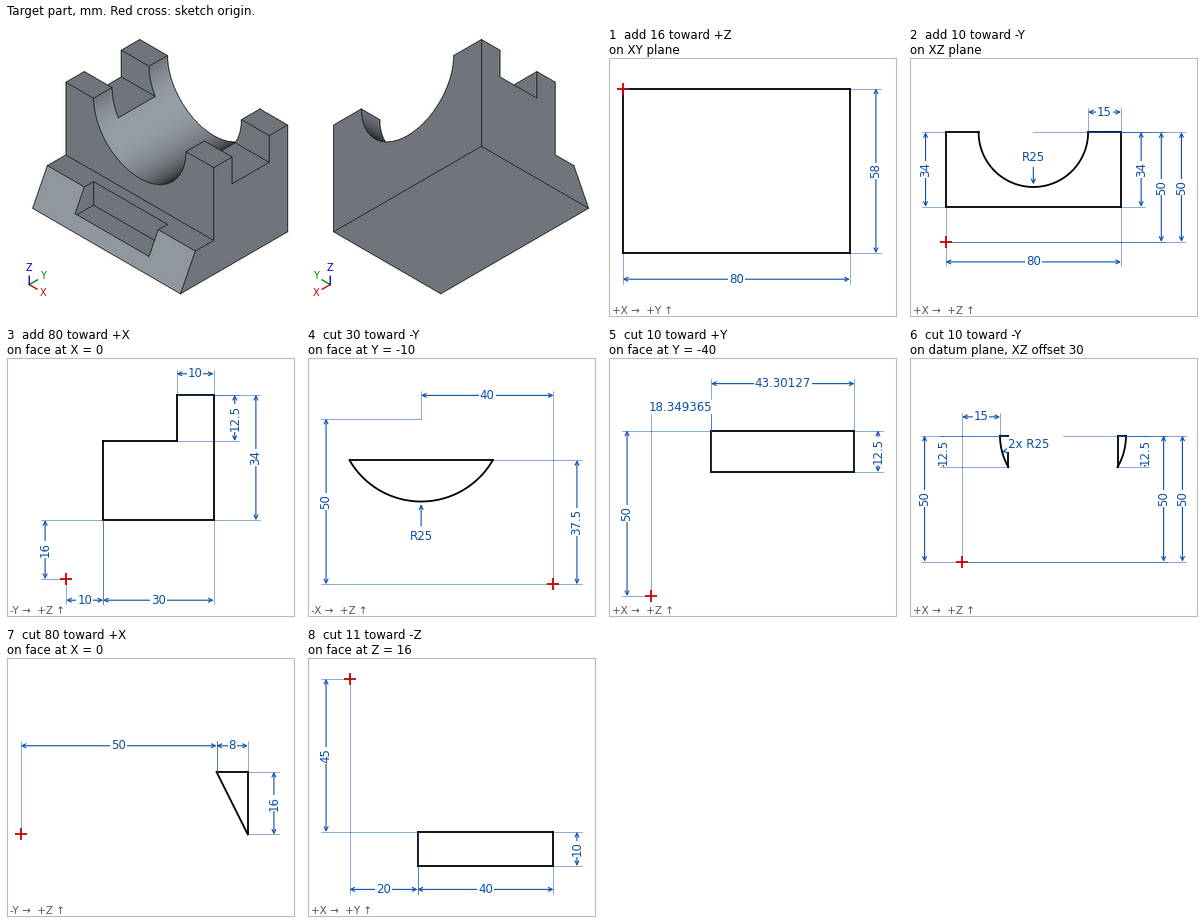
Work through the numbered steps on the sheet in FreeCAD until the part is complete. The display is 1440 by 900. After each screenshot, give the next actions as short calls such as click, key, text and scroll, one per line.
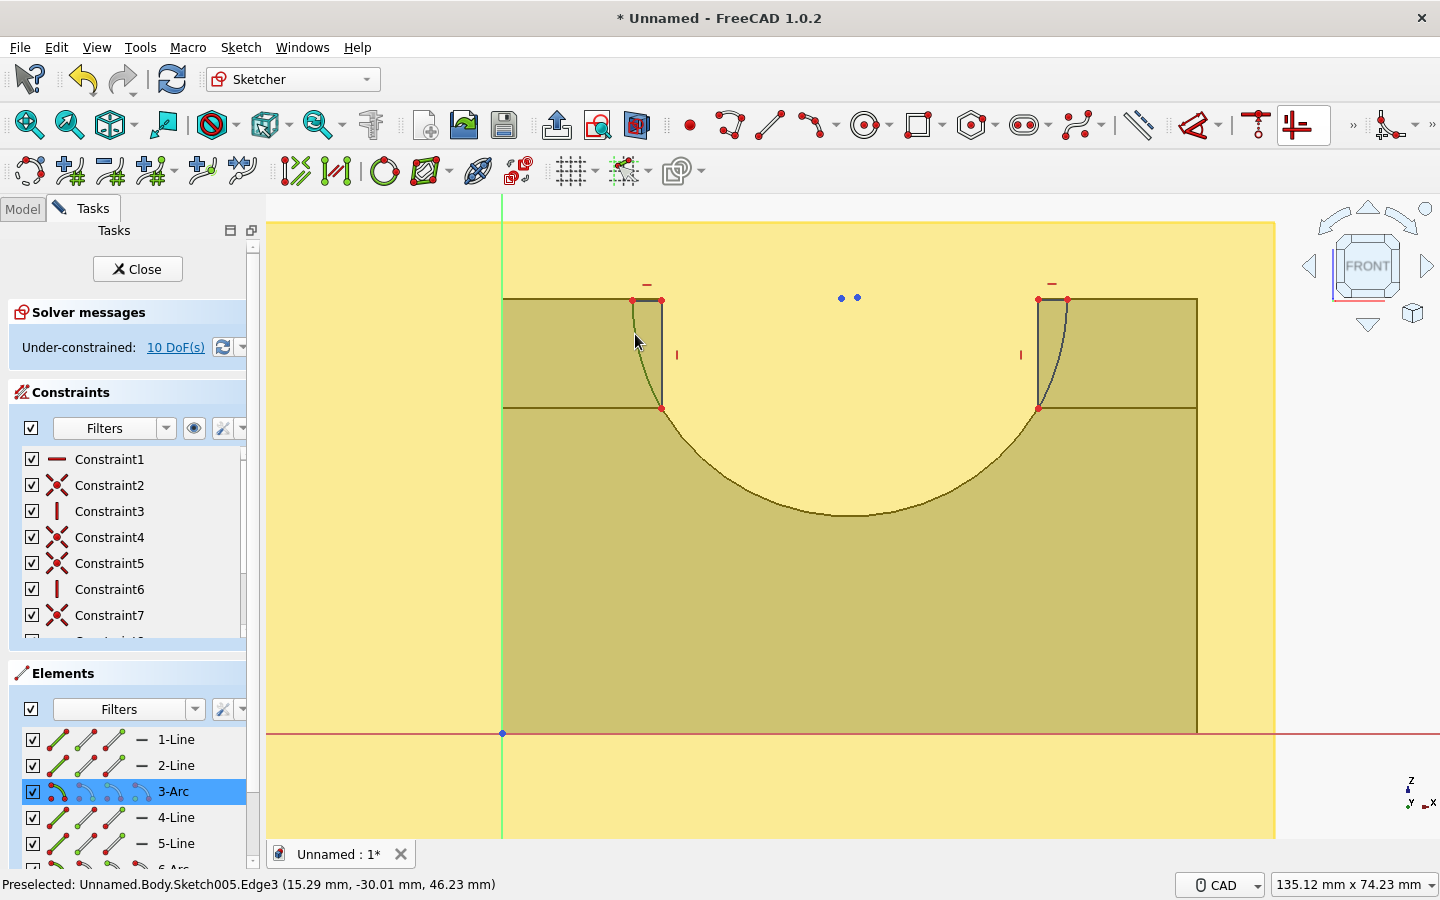
click(1052, 378)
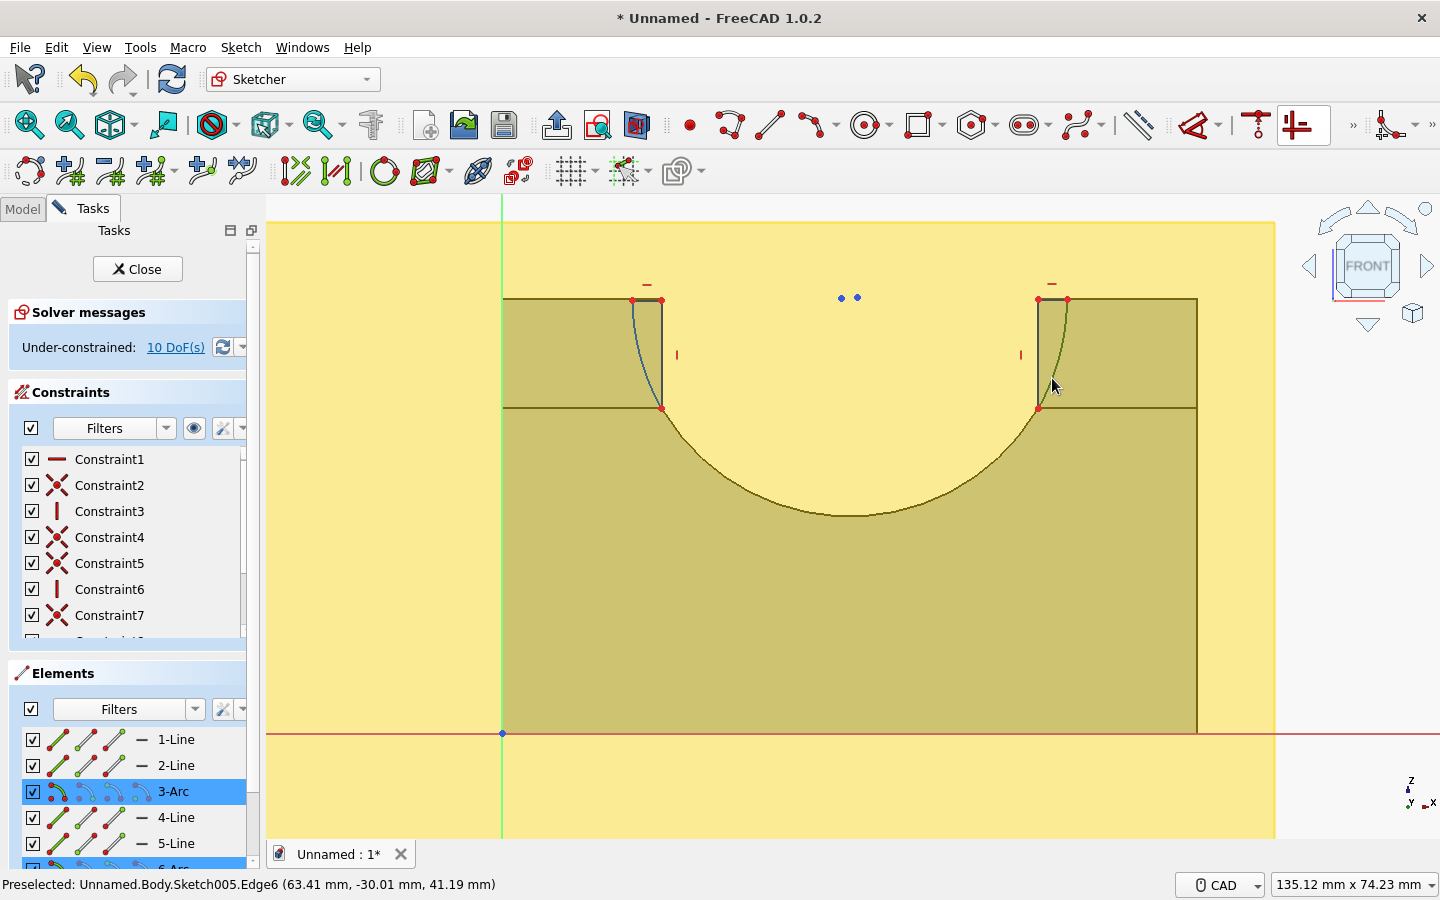
click(1256, 126)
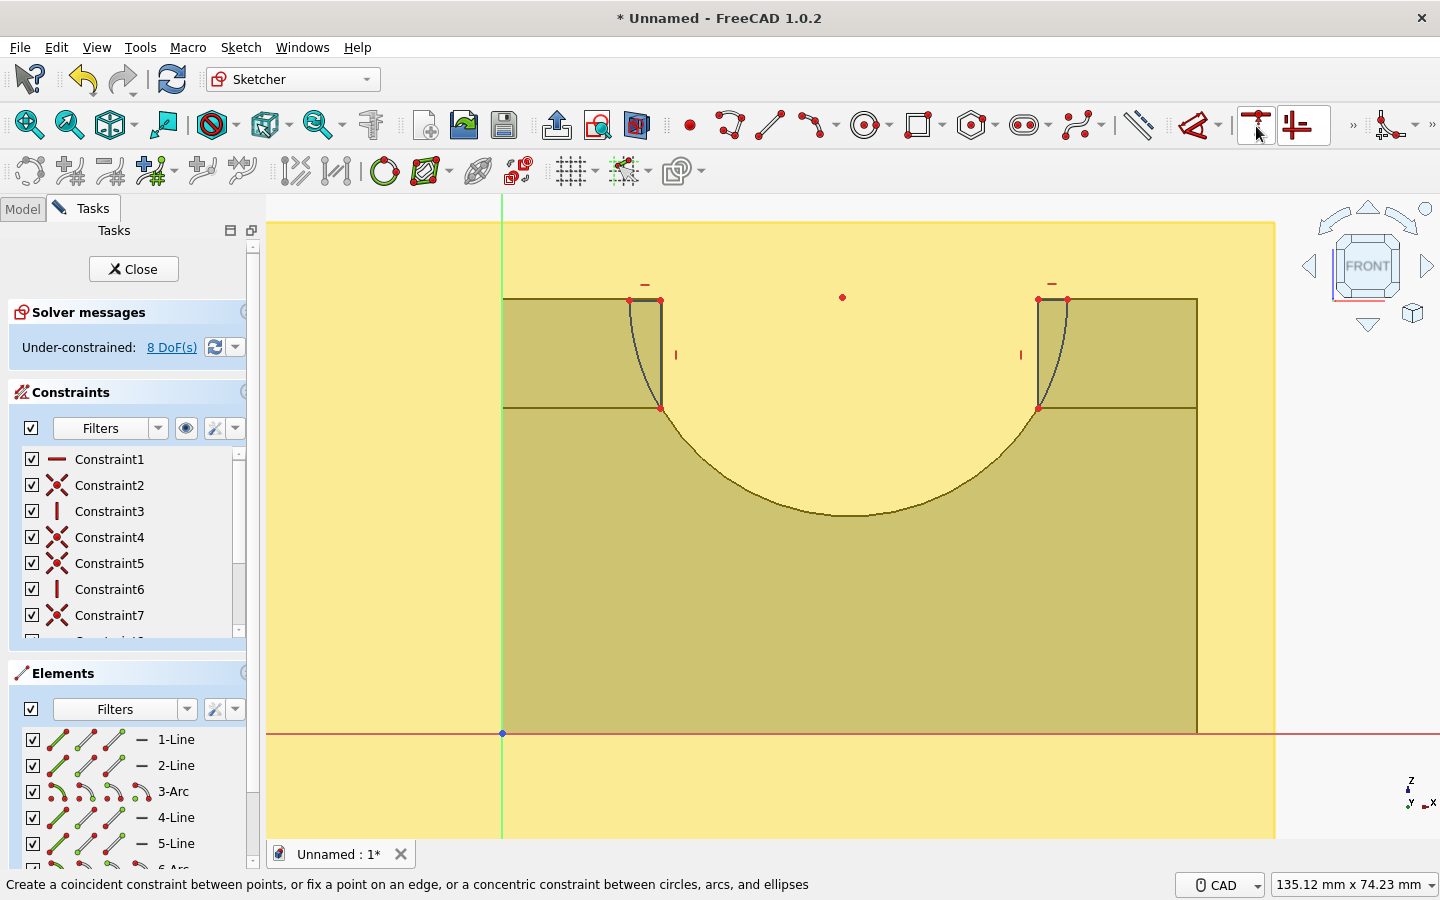
click(633, 335)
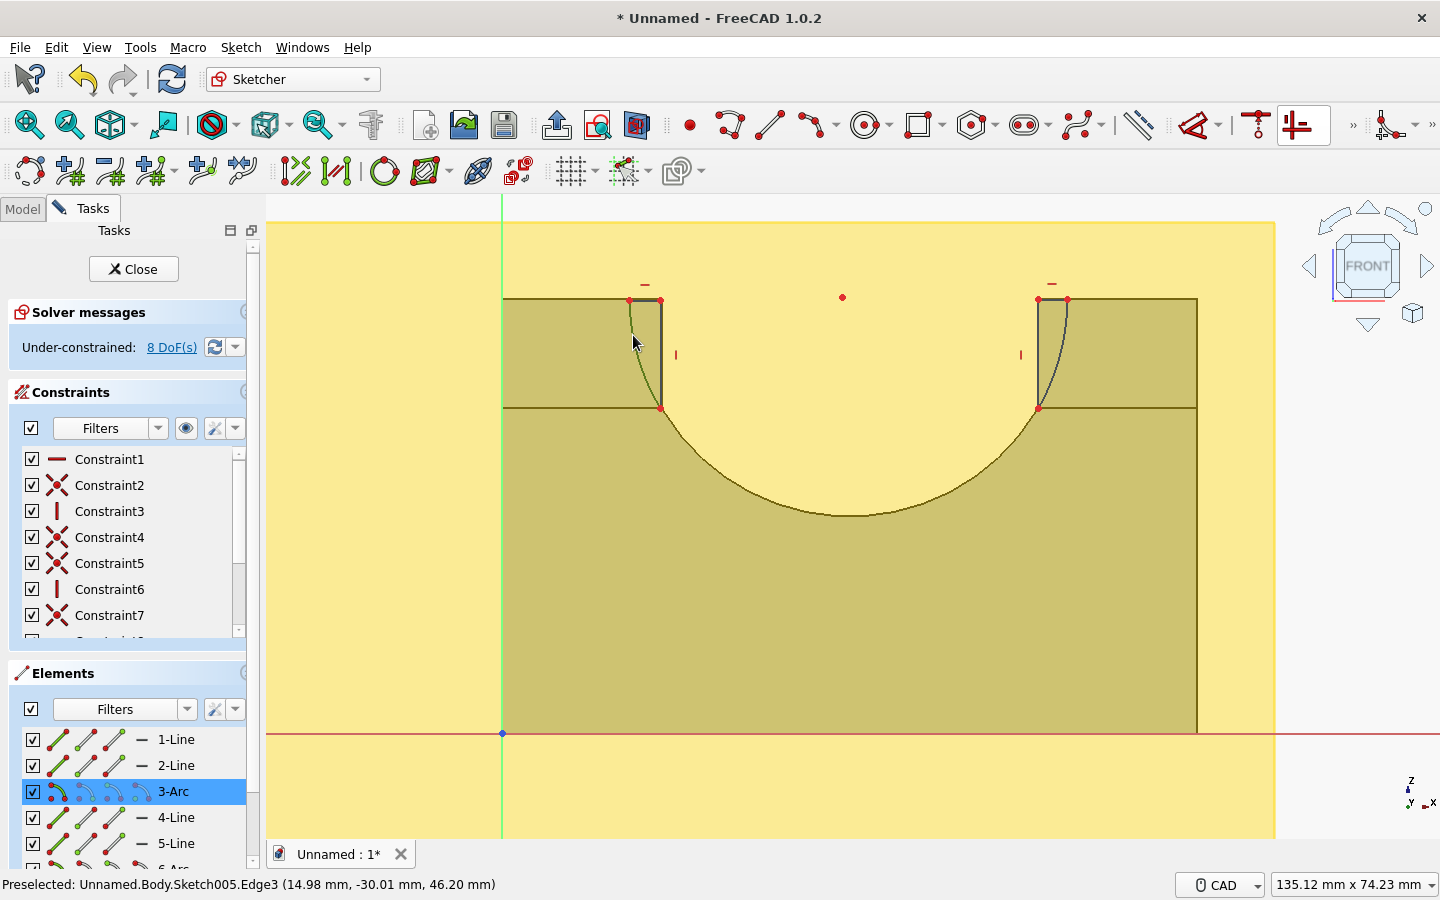
click(1053, 378)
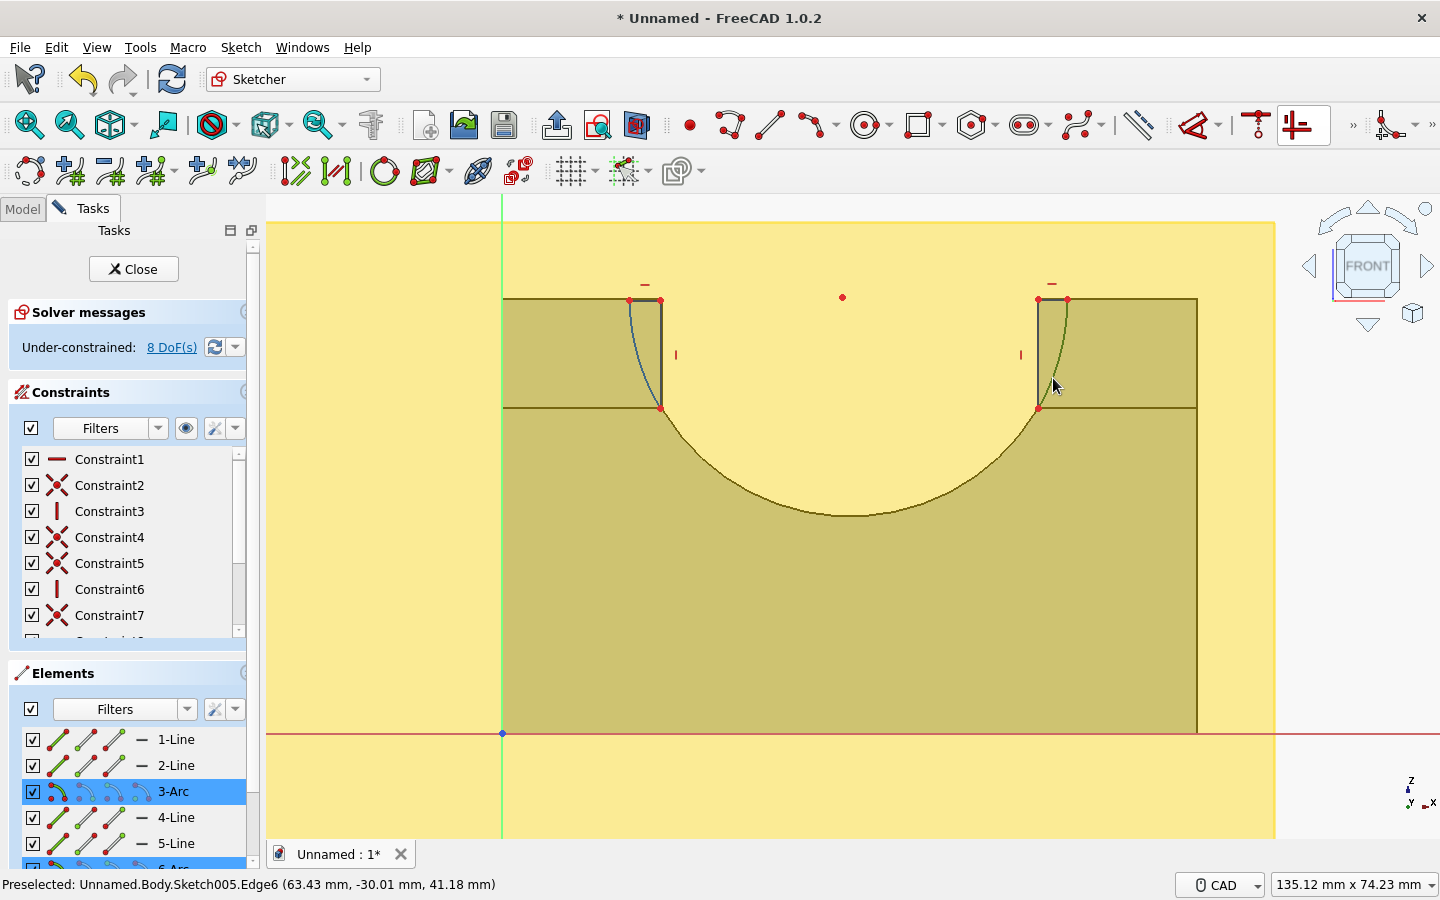
key(e)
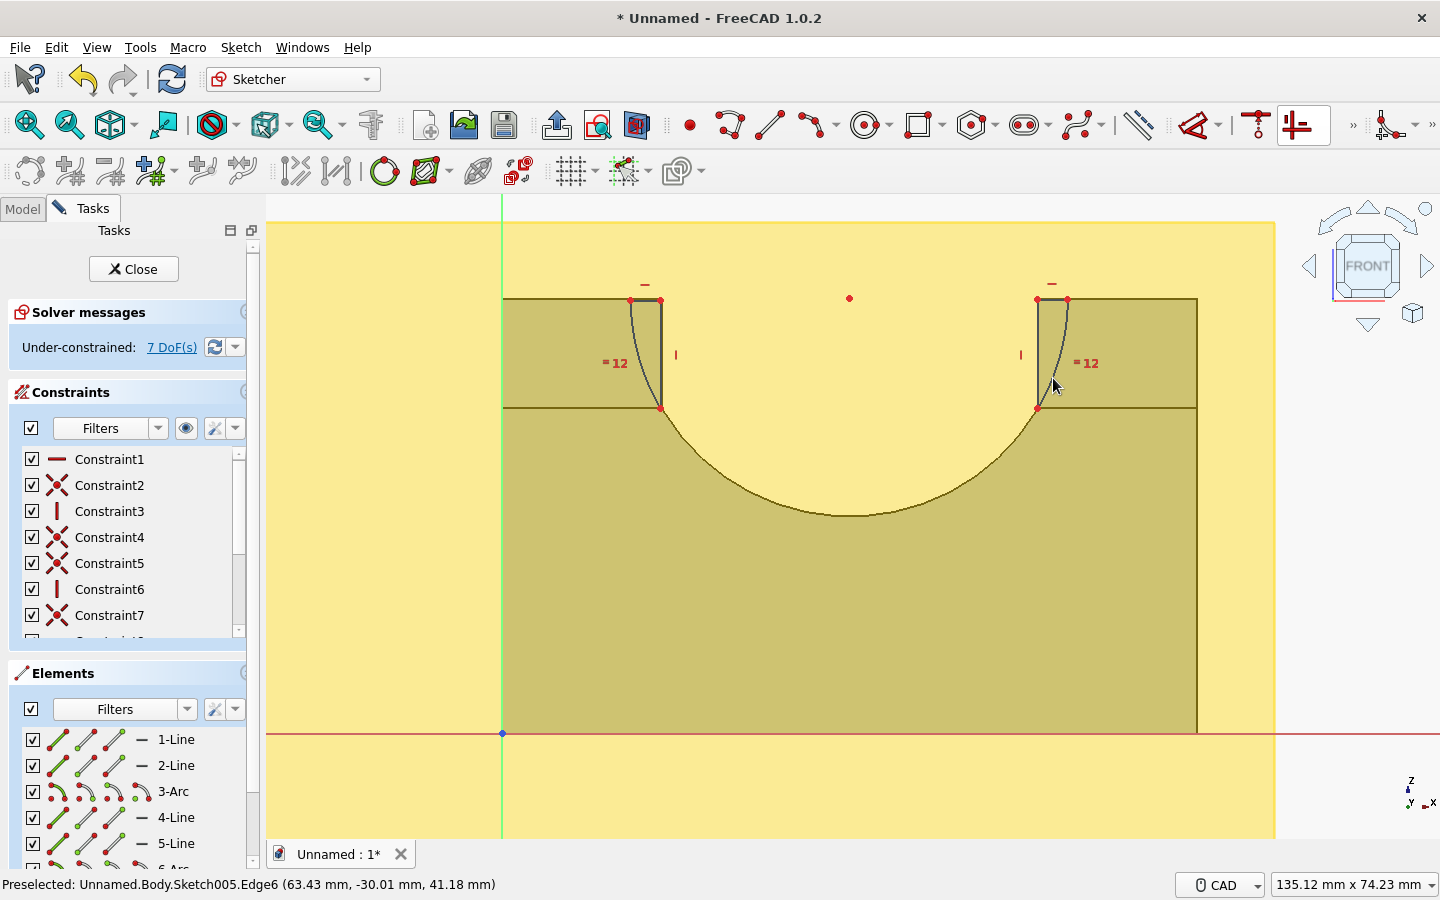
click(1194, 126)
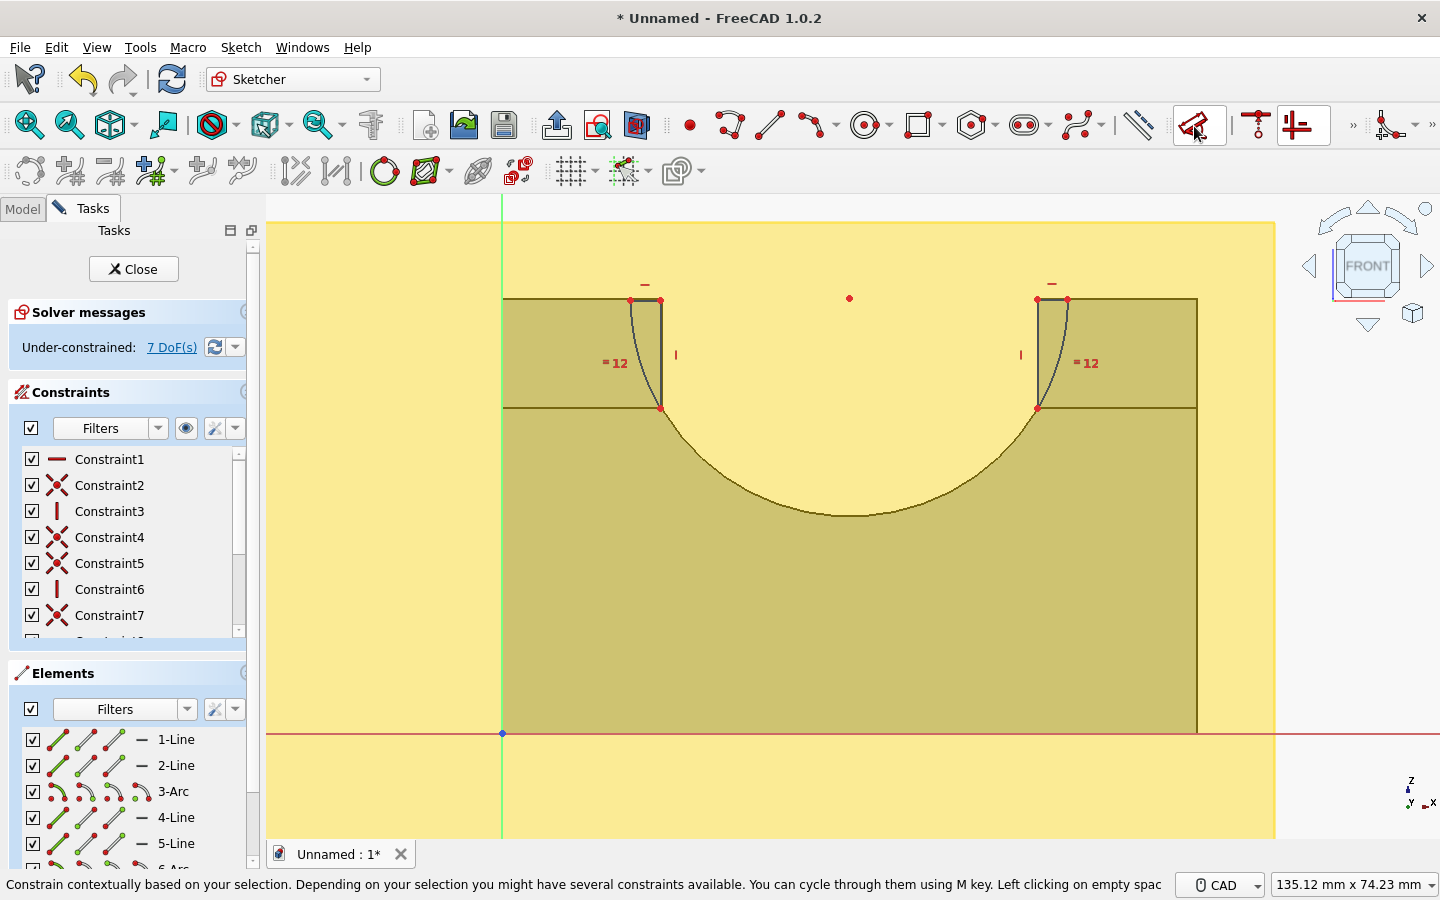
click(634, 335)
click(602, 340)